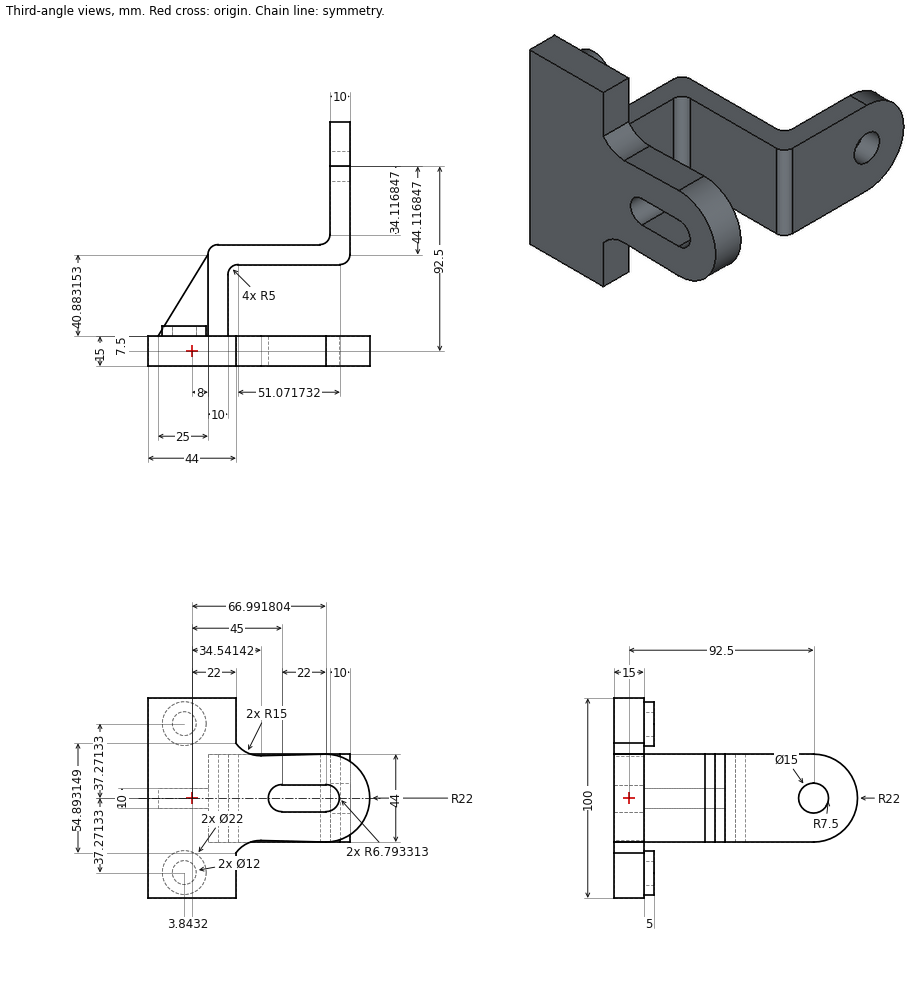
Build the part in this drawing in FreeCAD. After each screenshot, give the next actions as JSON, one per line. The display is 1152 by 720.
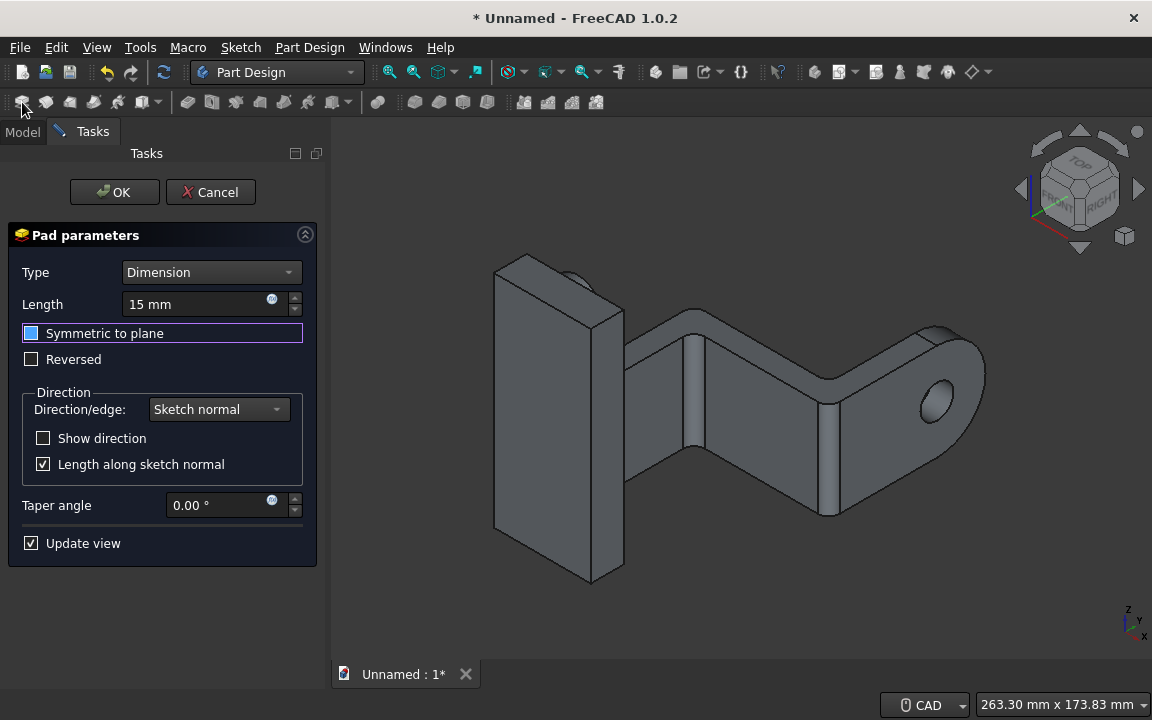
{"action": "left_click", "coordinate": [30, 359]}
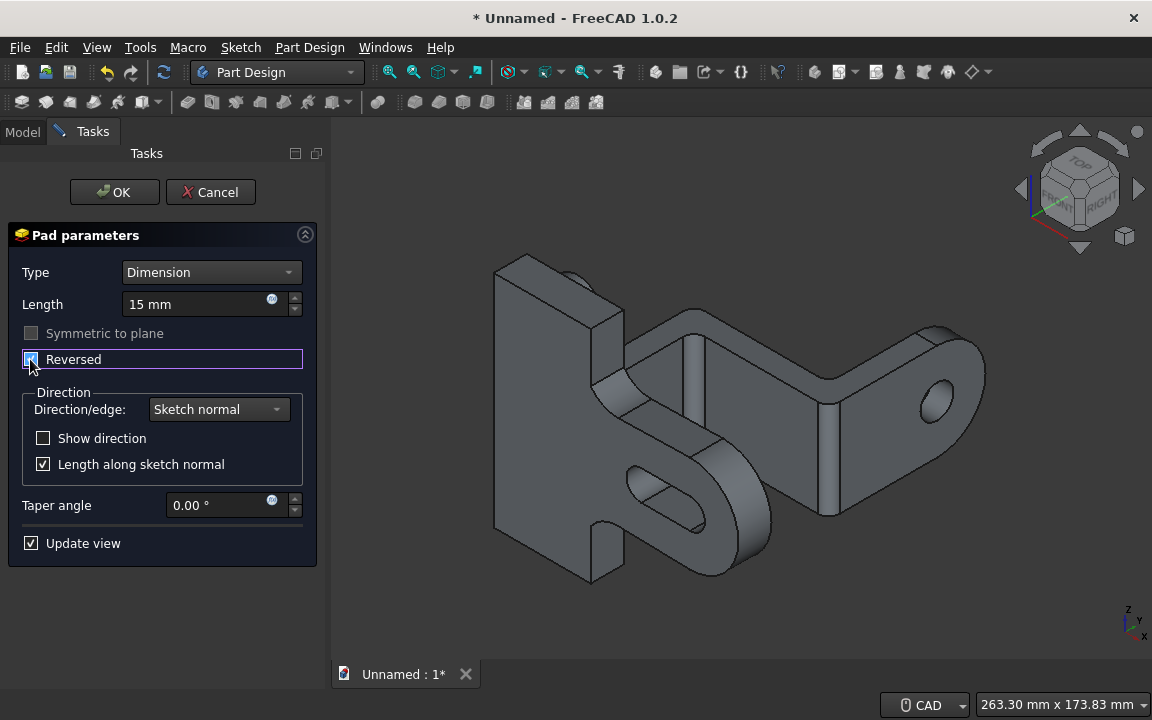
{"action": "left_click", "coordinate": [115, 192]}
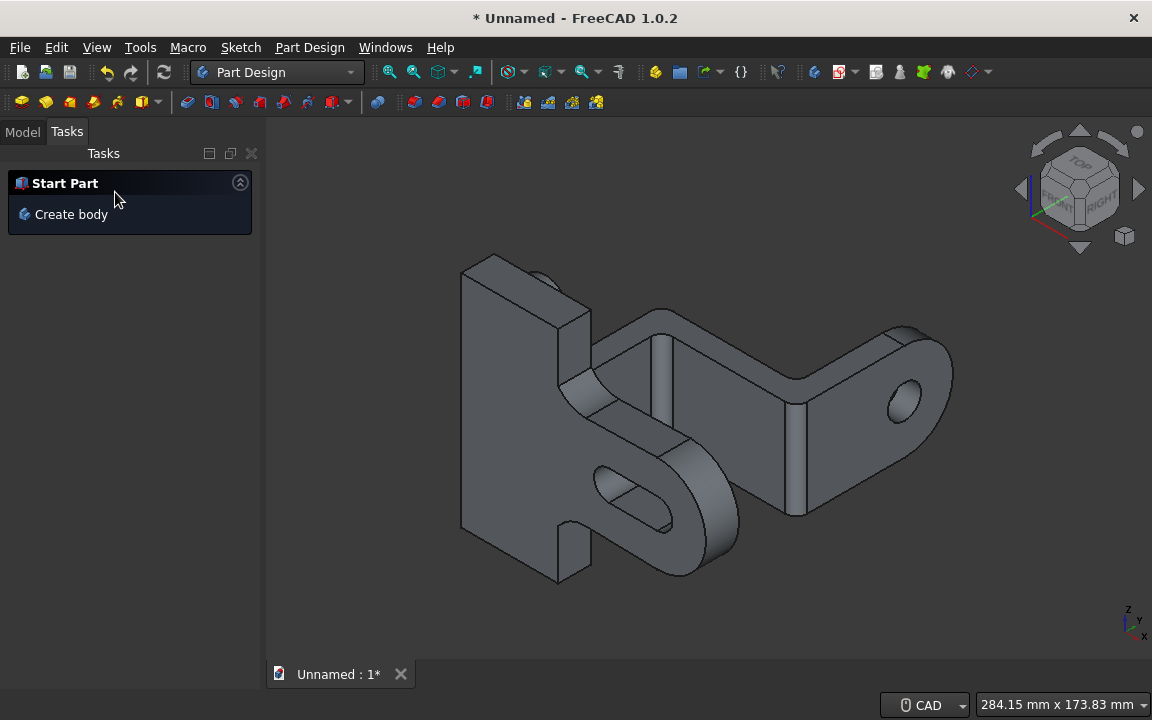
{"action": "left_click", "coordinate": [390, 72]}